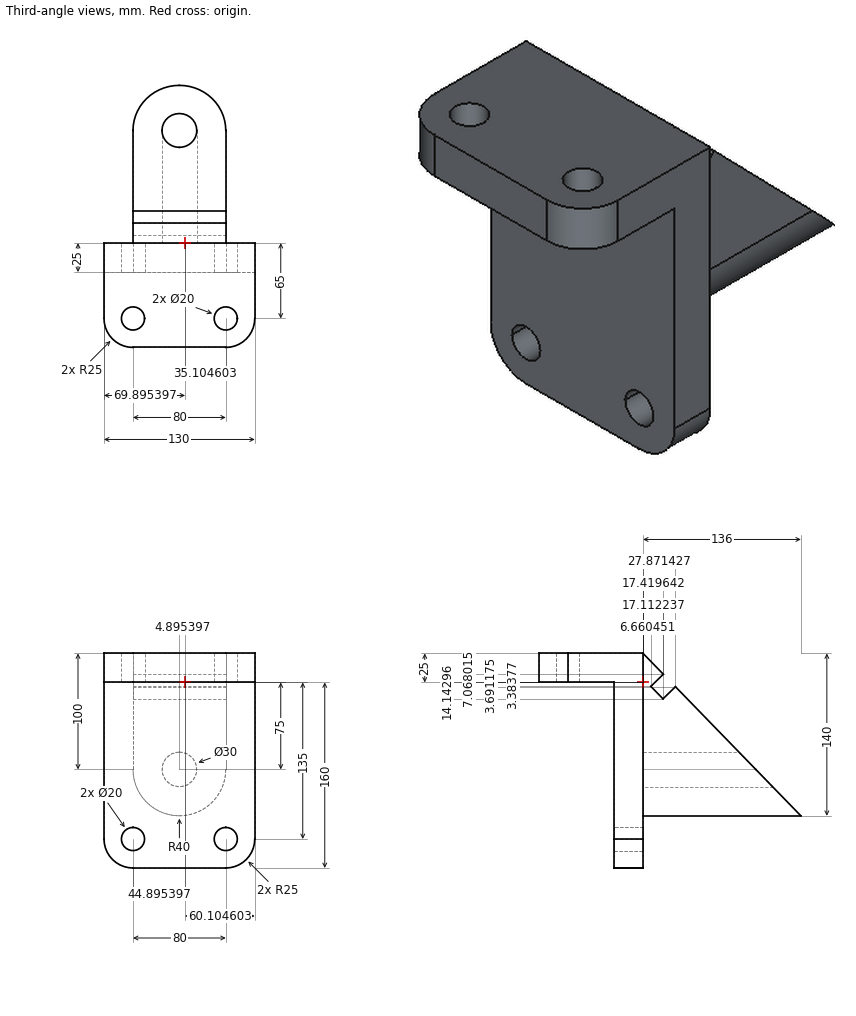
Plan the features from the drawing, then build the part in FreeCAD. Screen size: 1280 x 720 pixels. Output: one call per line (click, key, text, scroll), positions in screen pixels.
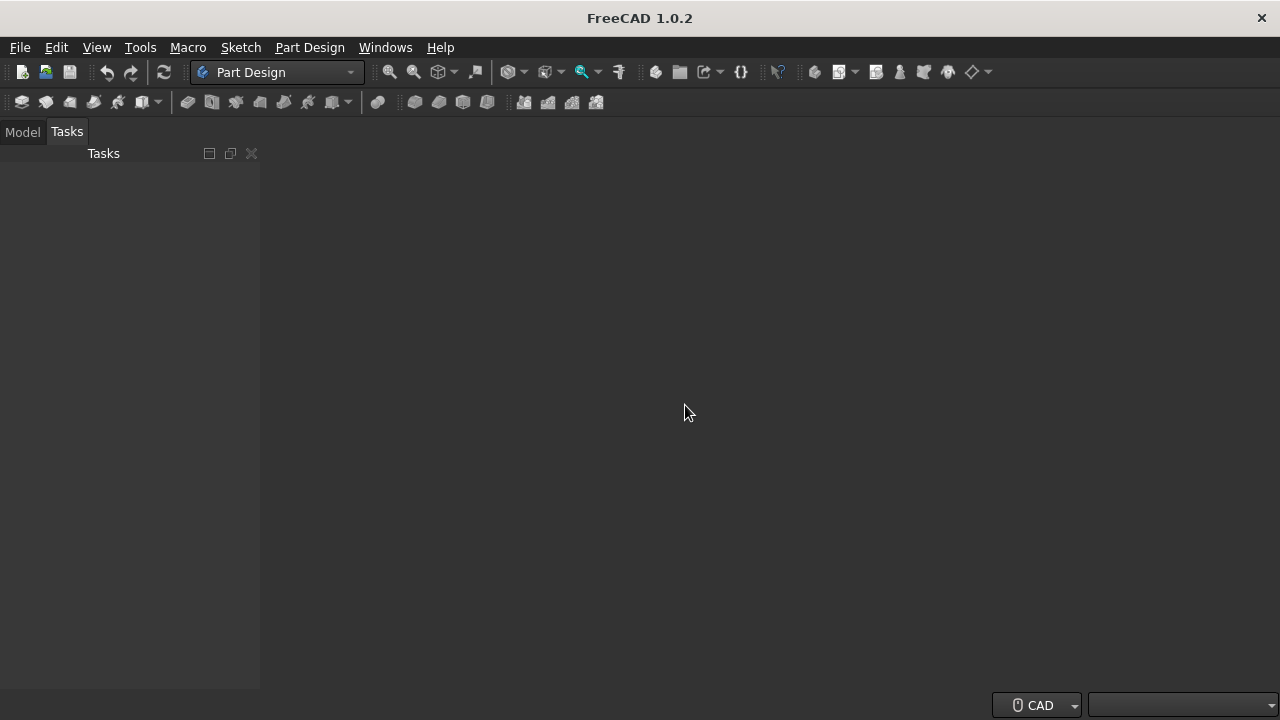
click(22, 72)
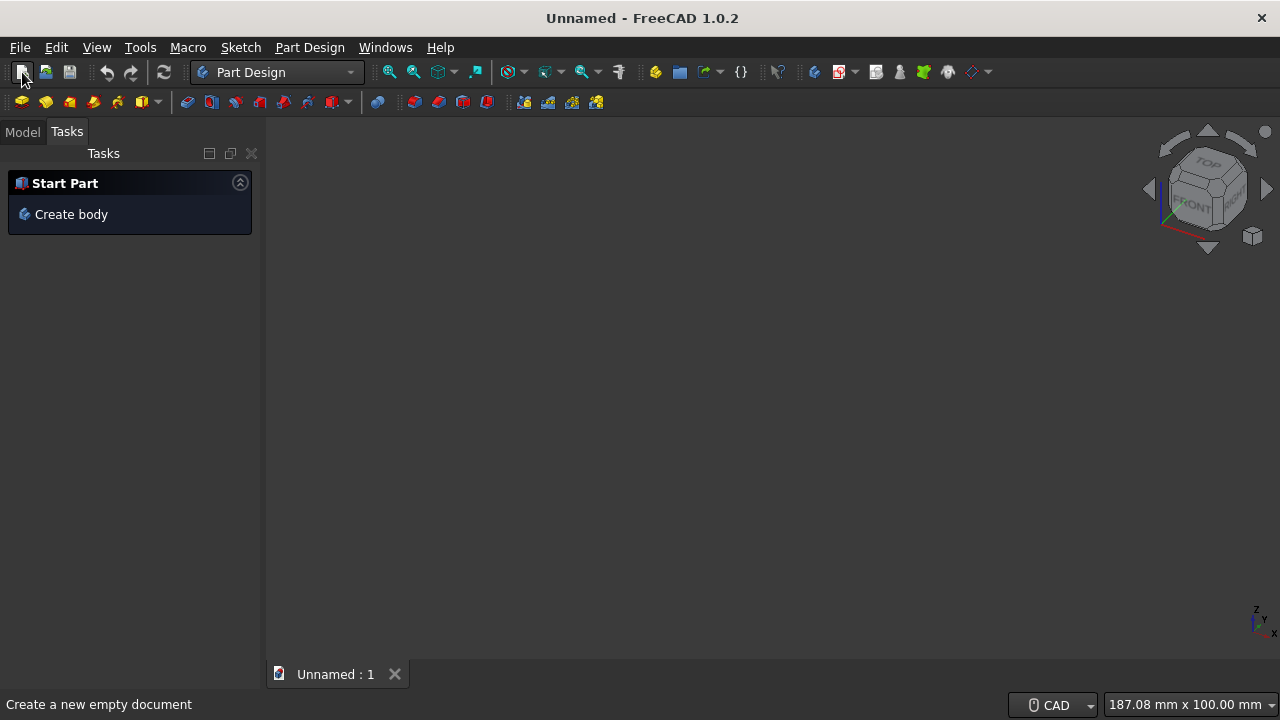
click(840, 72)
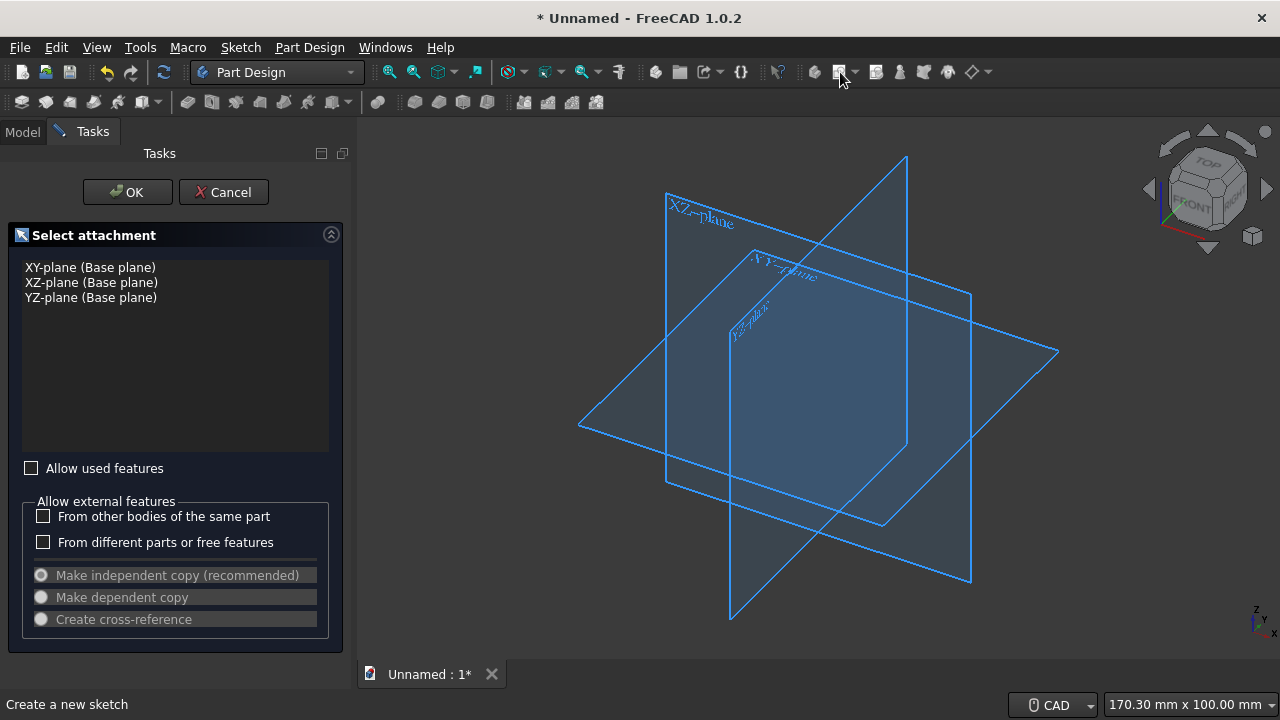
click(82, 268)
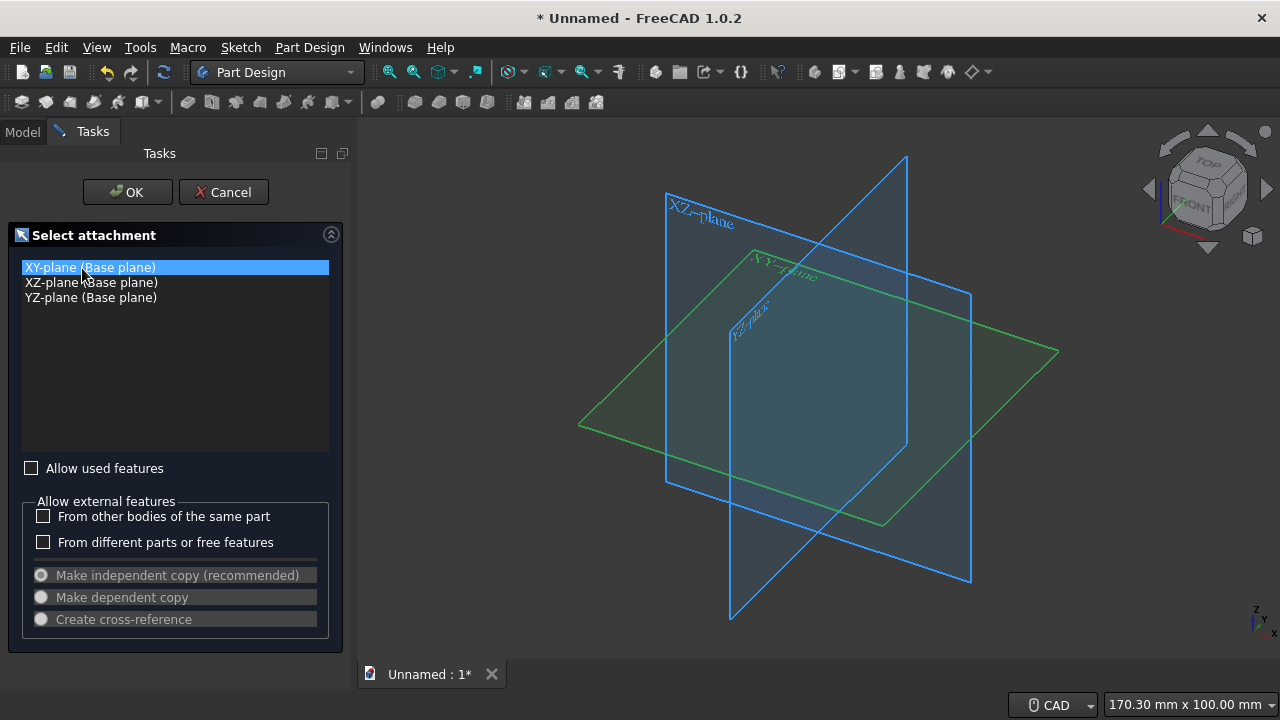
click(128, 192)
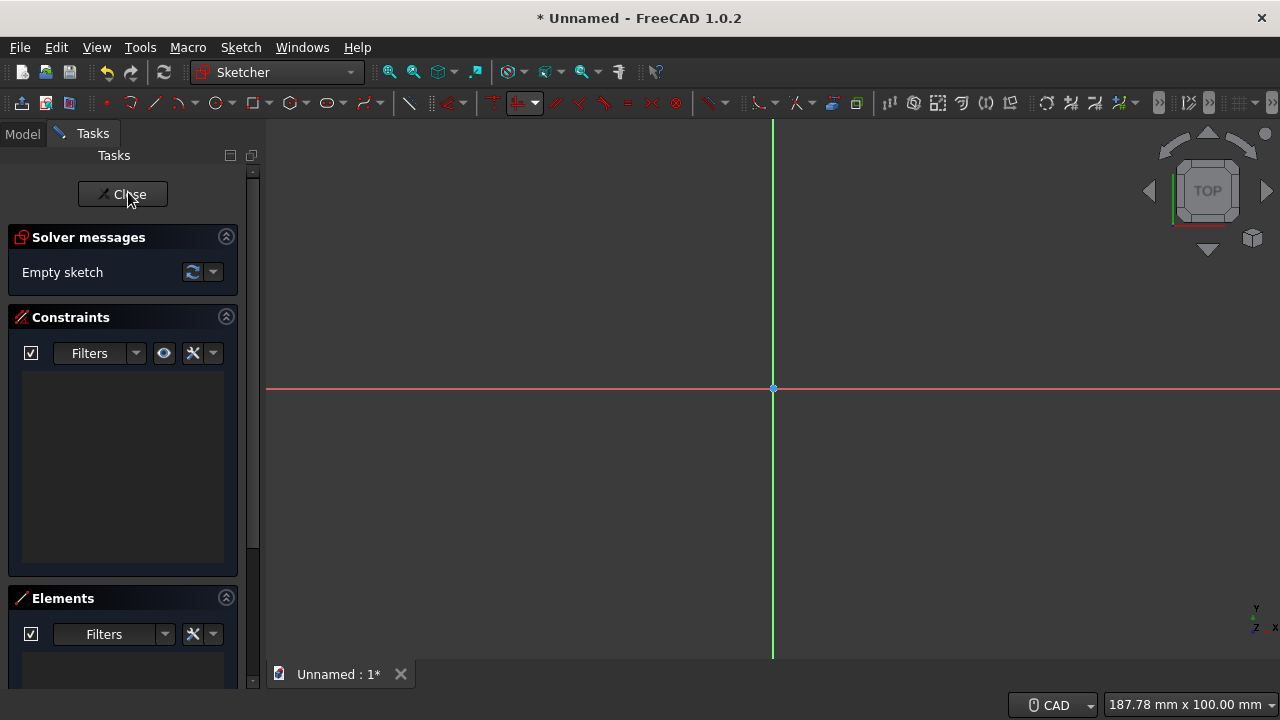
scroll(653, 147, down, 3)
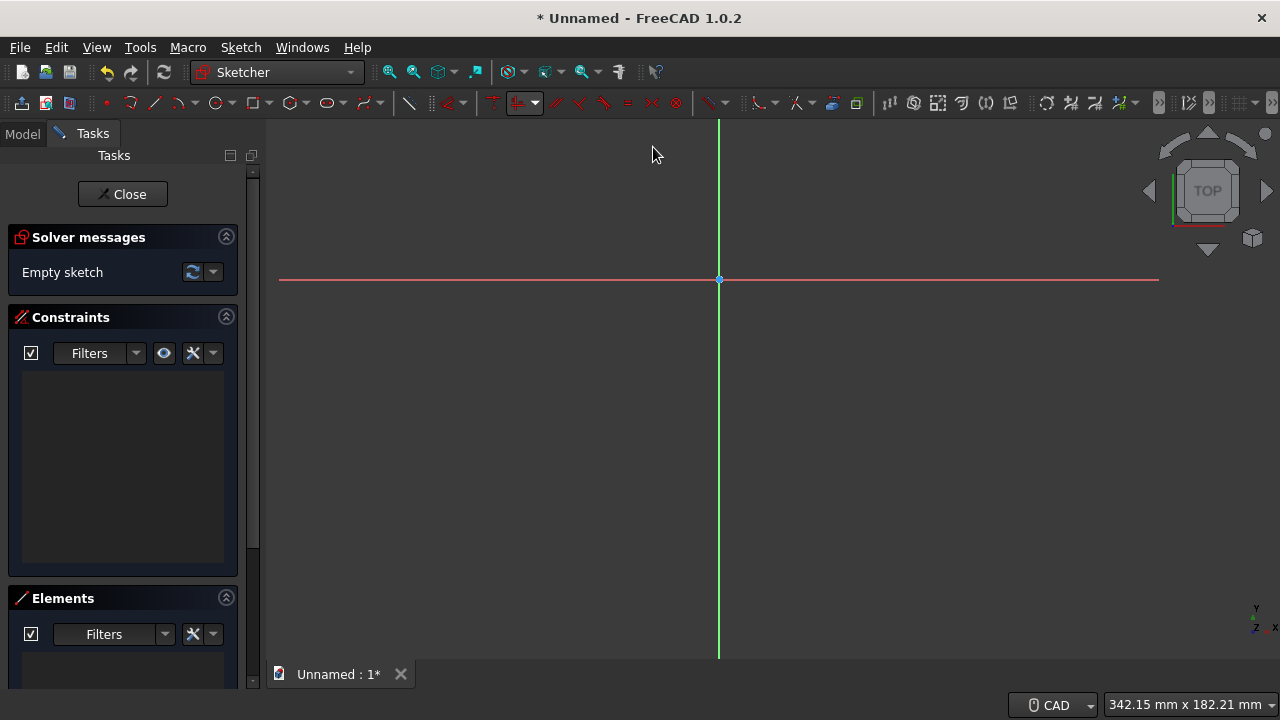
click(156, 104)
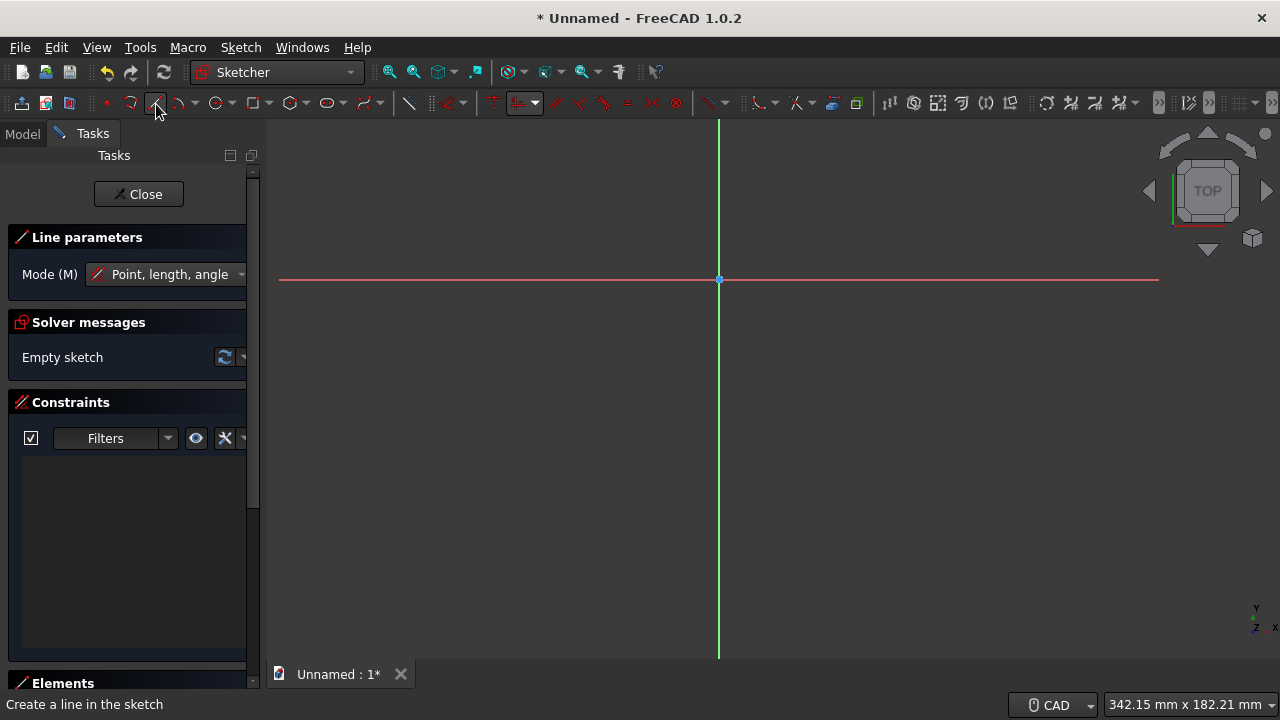
click(586, 547)
click(823, 547)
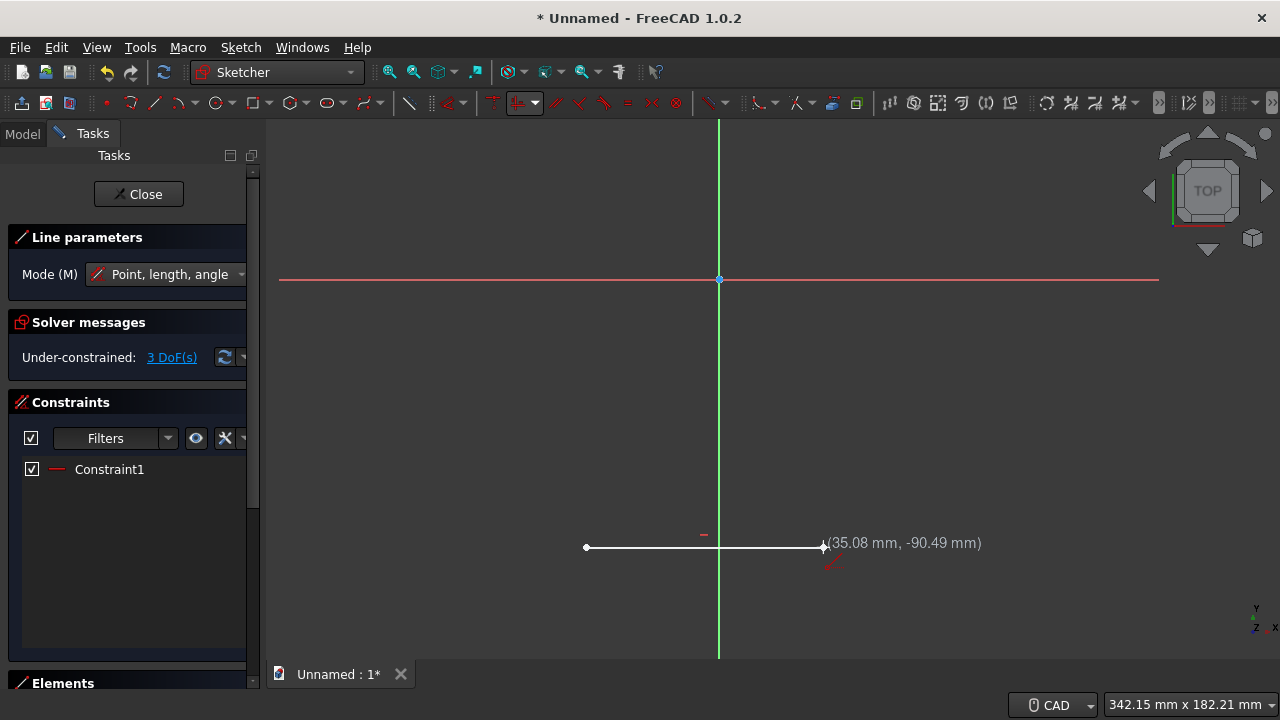
key(g)
key(m)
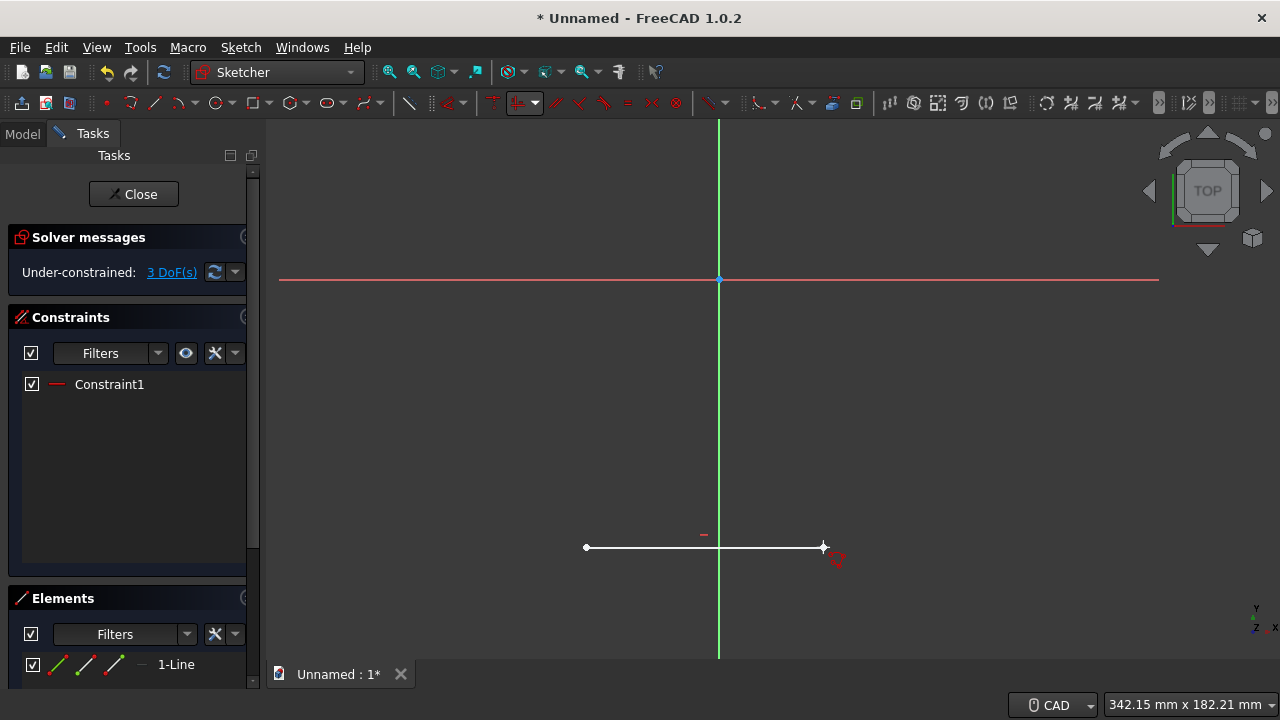
click(897, 472)
click(897, 280)
click(512, 289)
click(512, 472)
right_click(512, 472)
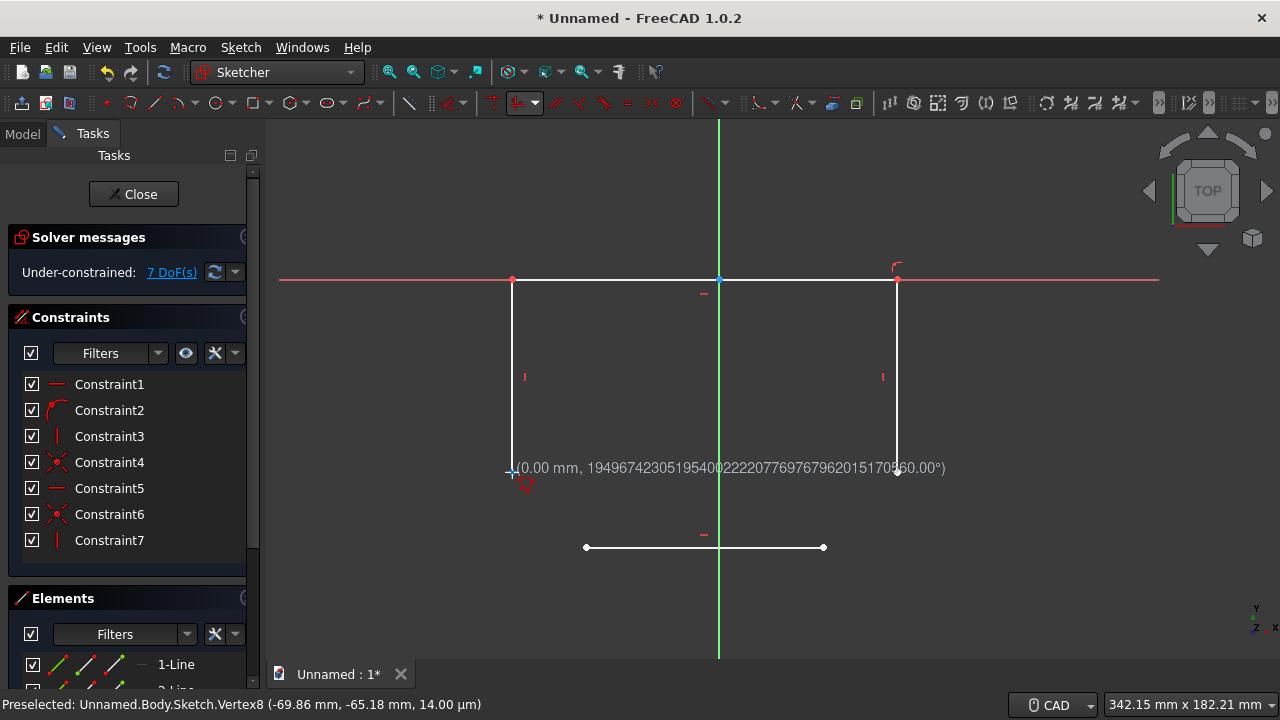
key(g)
key(3)
key(a)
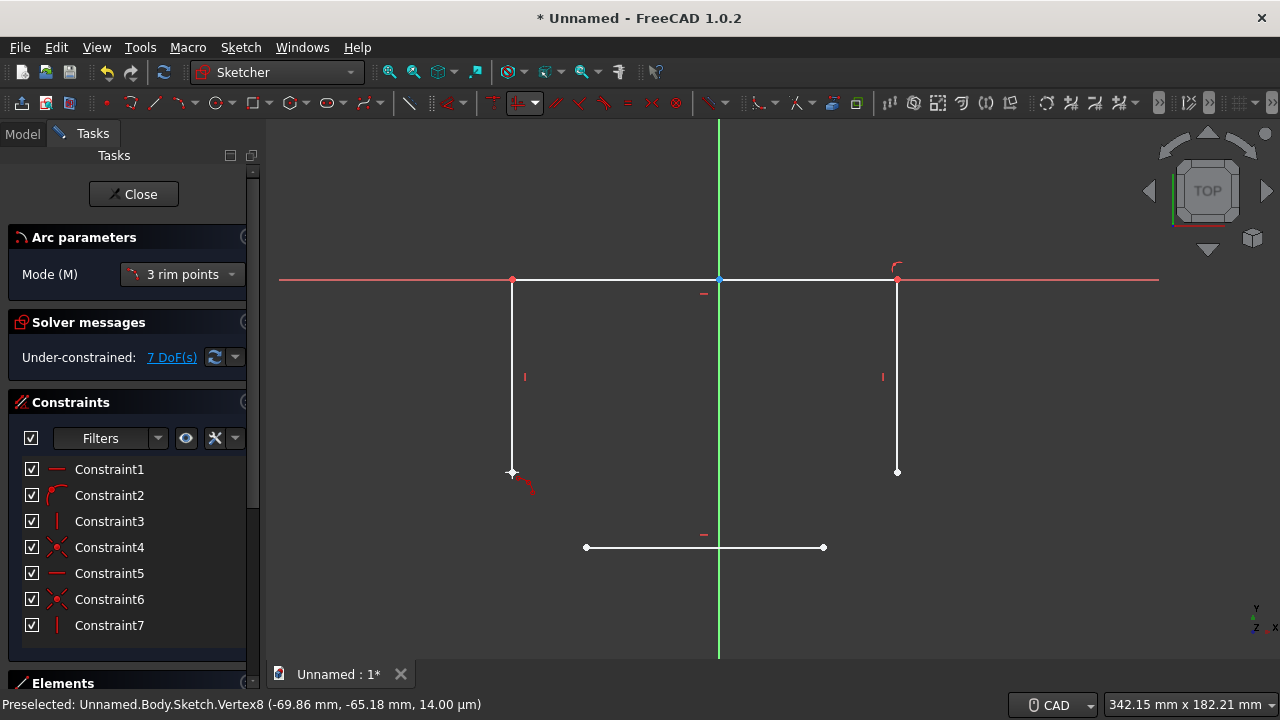
click(823, 548)
click(897, 473)
click(875, 525)